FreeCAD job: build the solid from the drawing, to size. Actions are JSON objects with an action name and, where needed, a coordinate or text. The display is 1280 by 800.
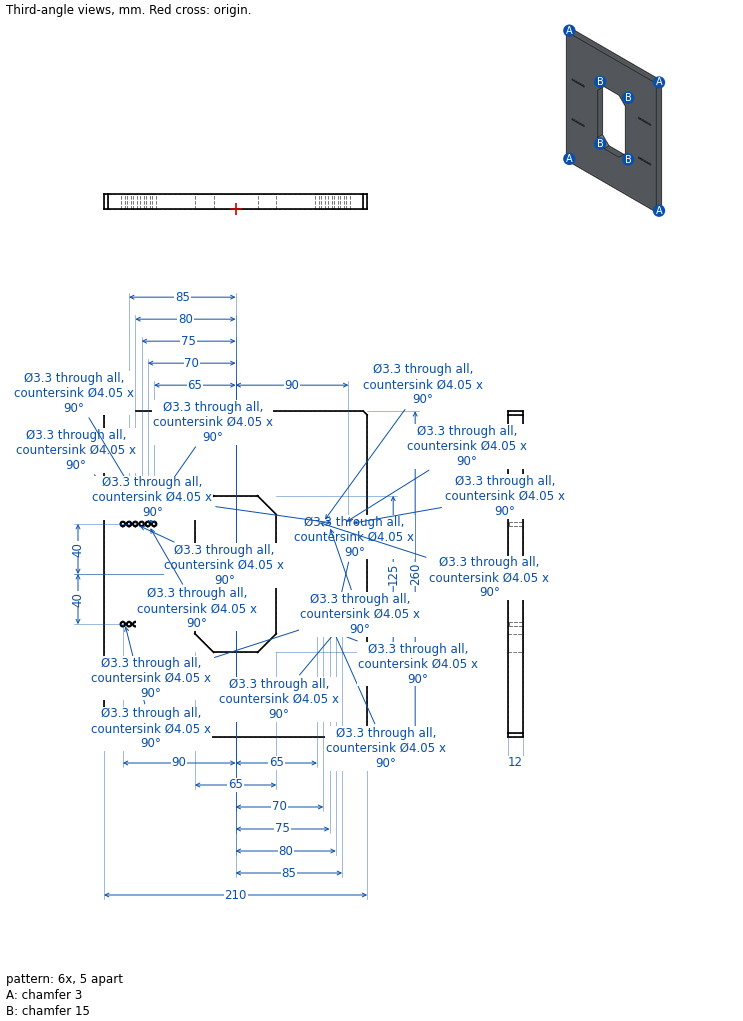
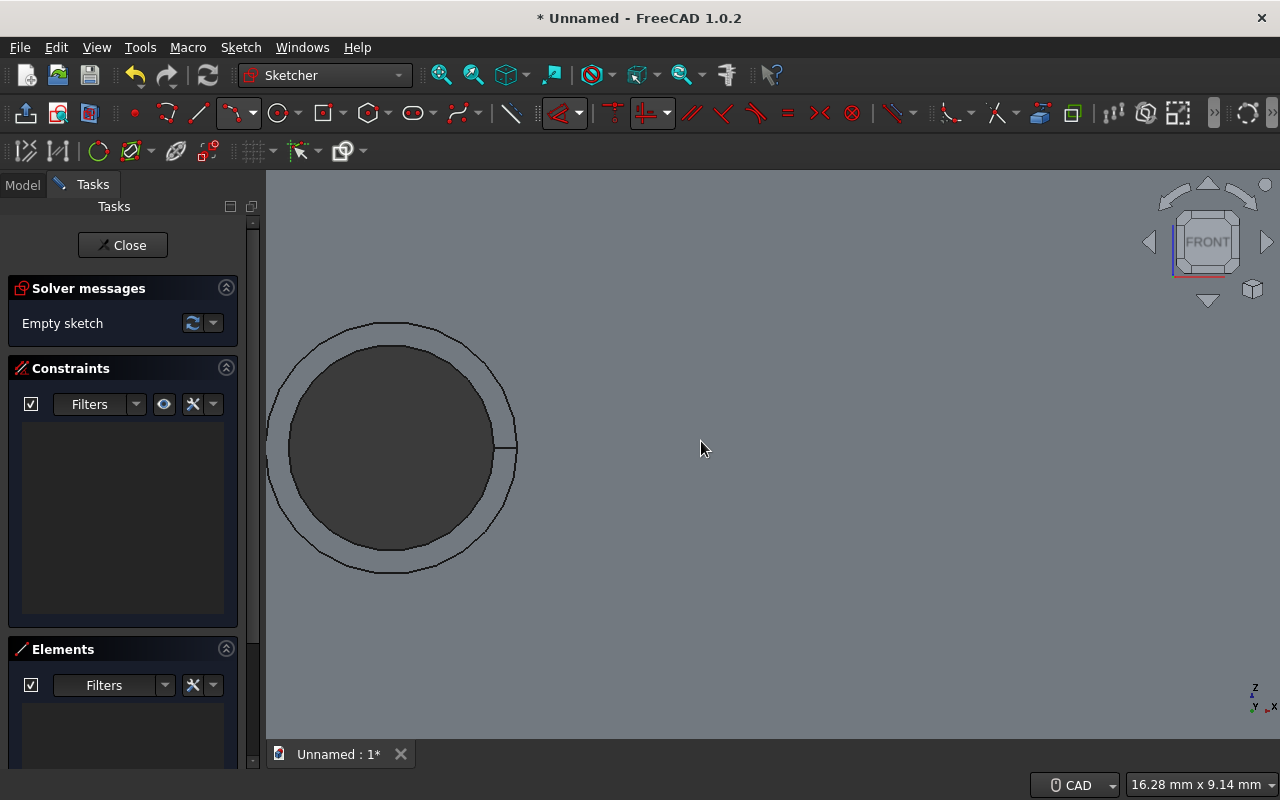
{"action": "left_click", "coordinate": [278, 114]}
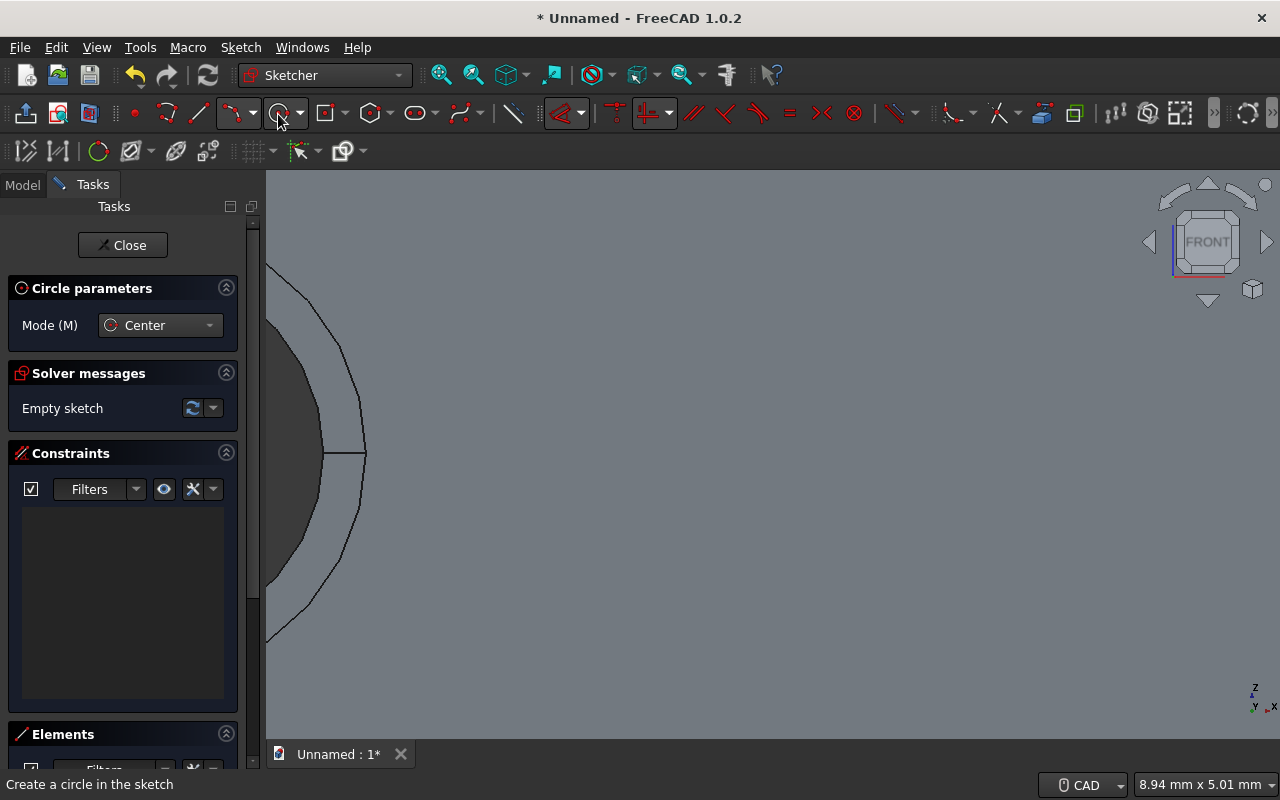
{"action": "left_click", "coordinate": [703, 453]}
{"action": "mouse_move", "coordinate": [836, 321]}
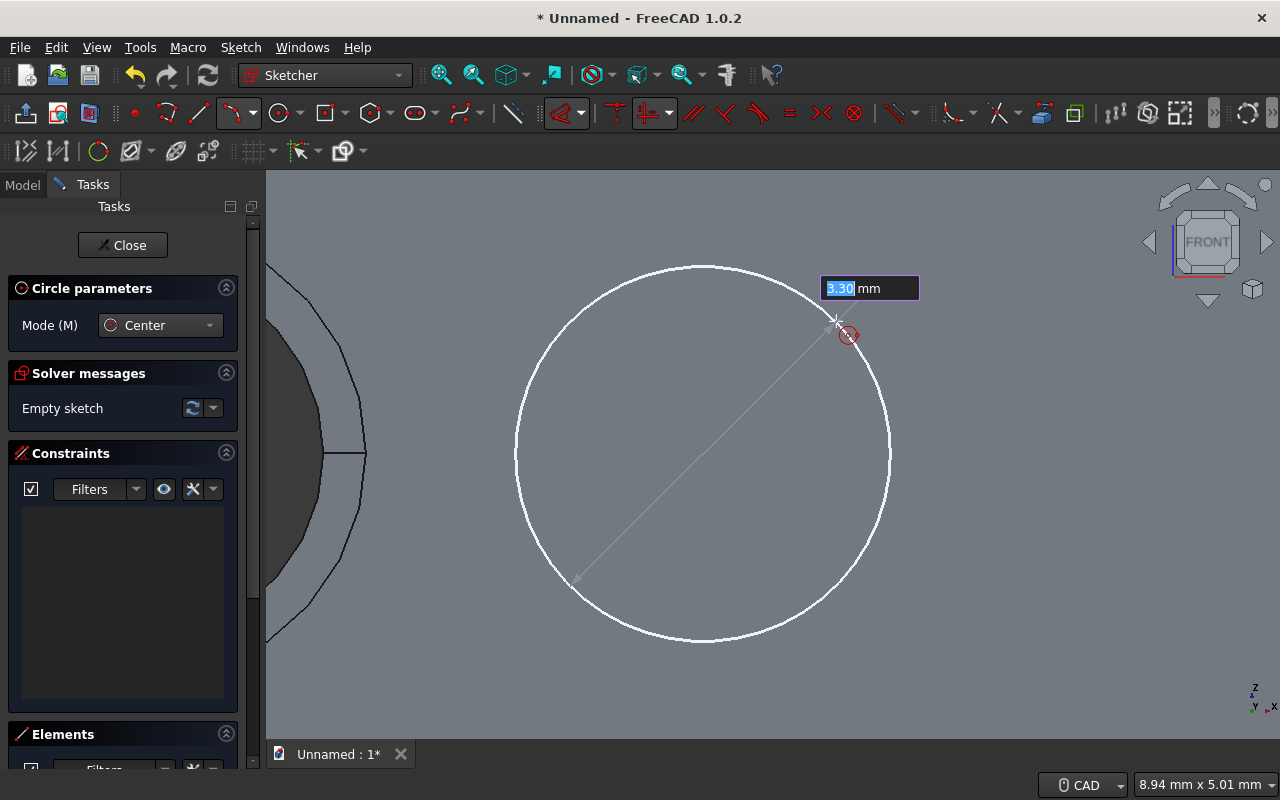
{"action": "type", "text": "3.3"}
{"action": "key", "text": "Return"}
{"action": "key", "text": "Escape"}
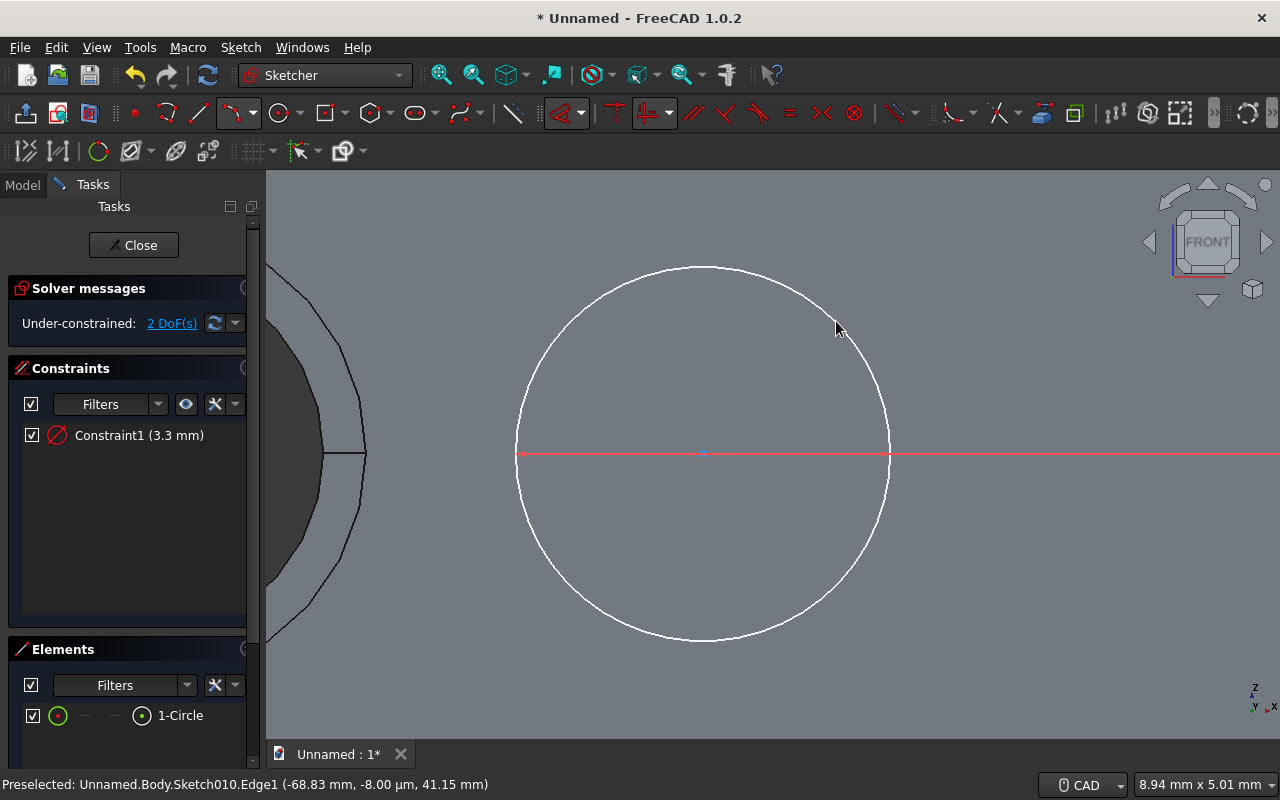
{"action": "left_click", "coordinate": [703, 454]}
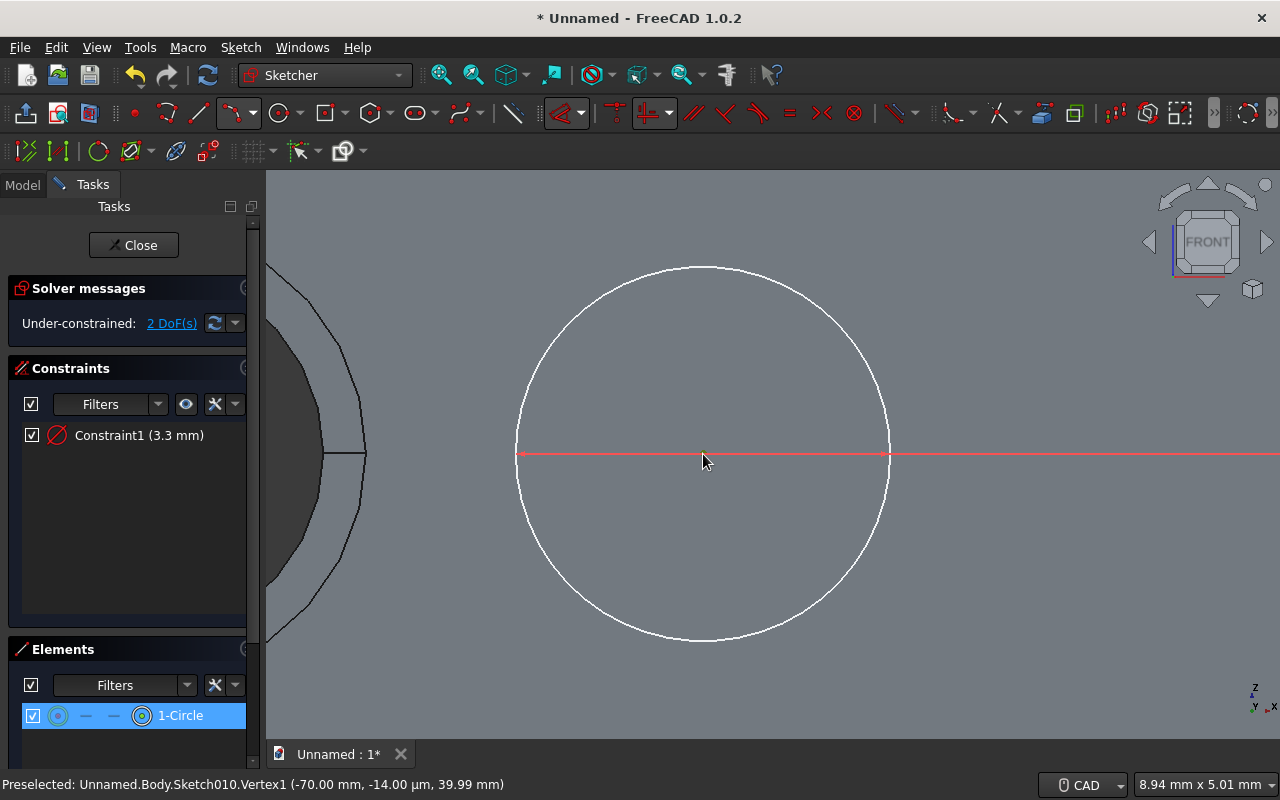
{"action": "left_click", "coordinate": [584, 114]}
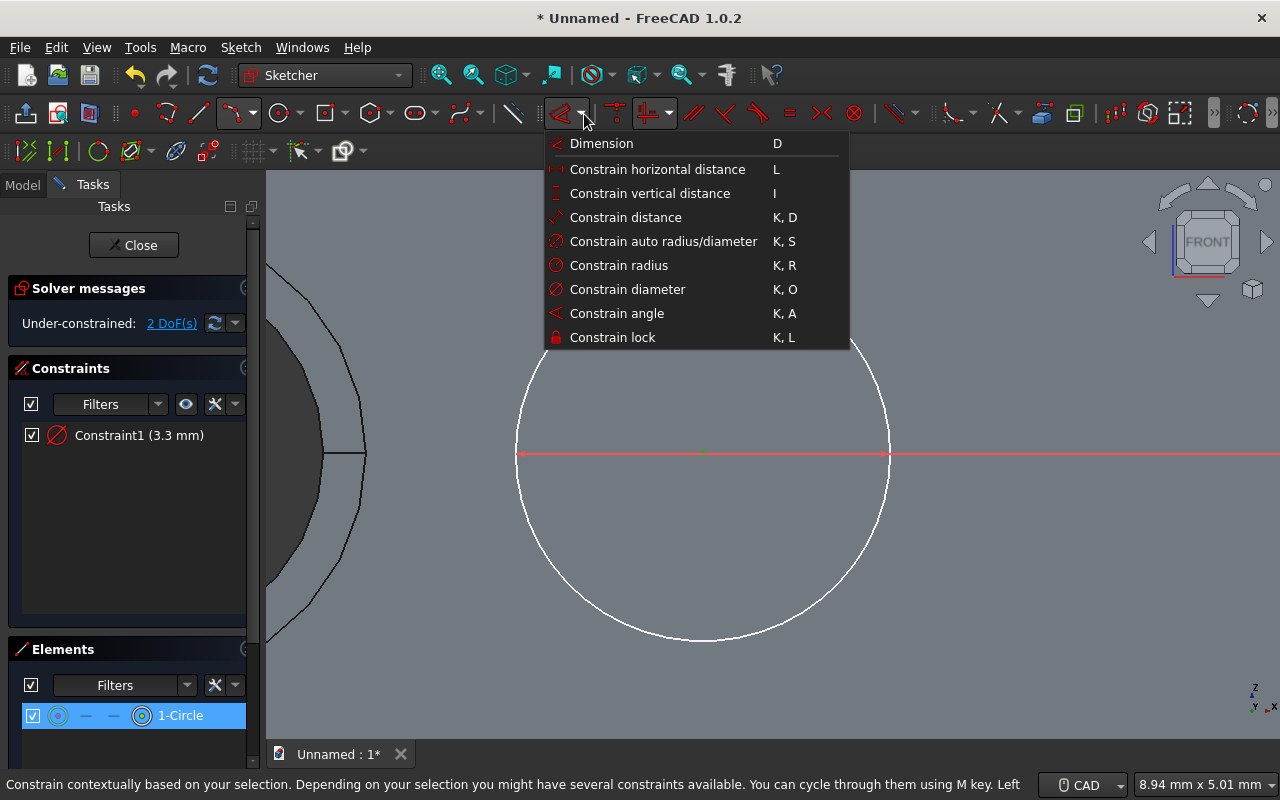
{"action": "left_click", "coordinate": [697, 169]}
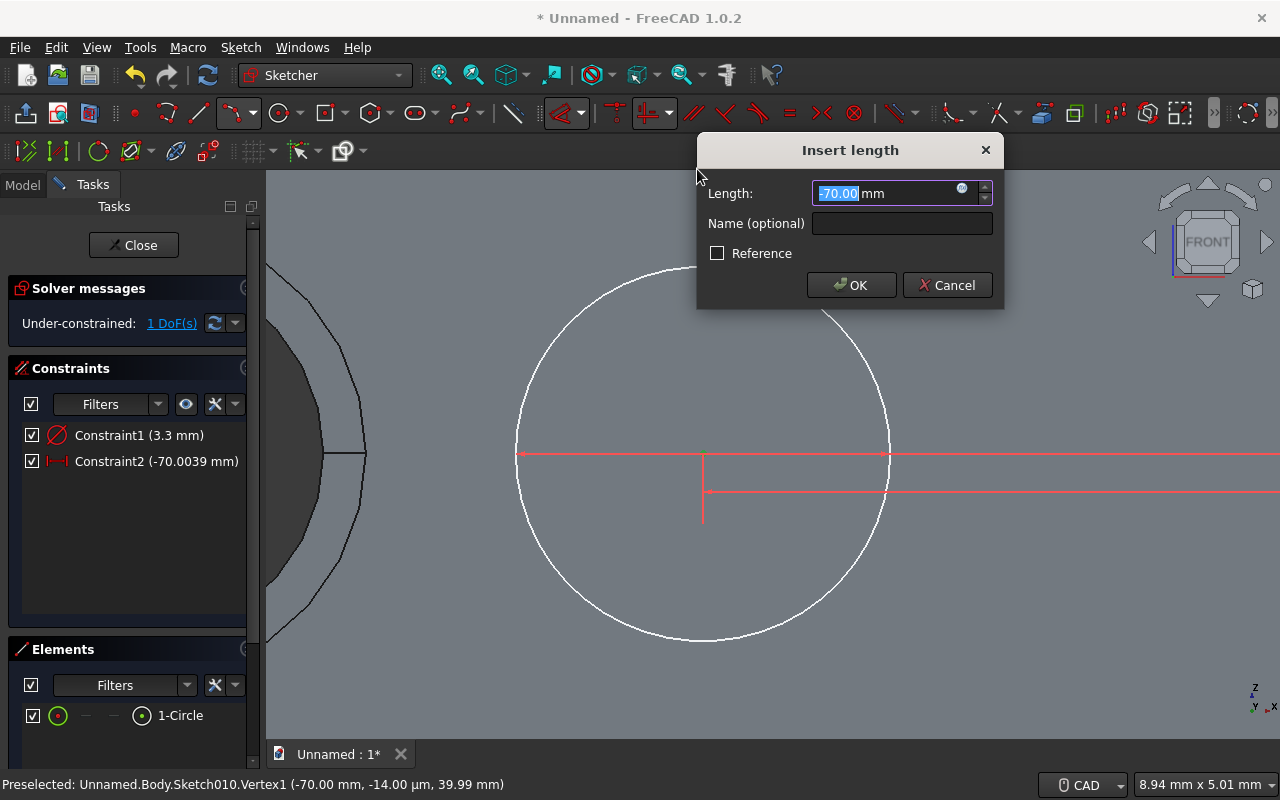
{"action": "type", "text": "-70"}
{"action": "key", "text": "Return"}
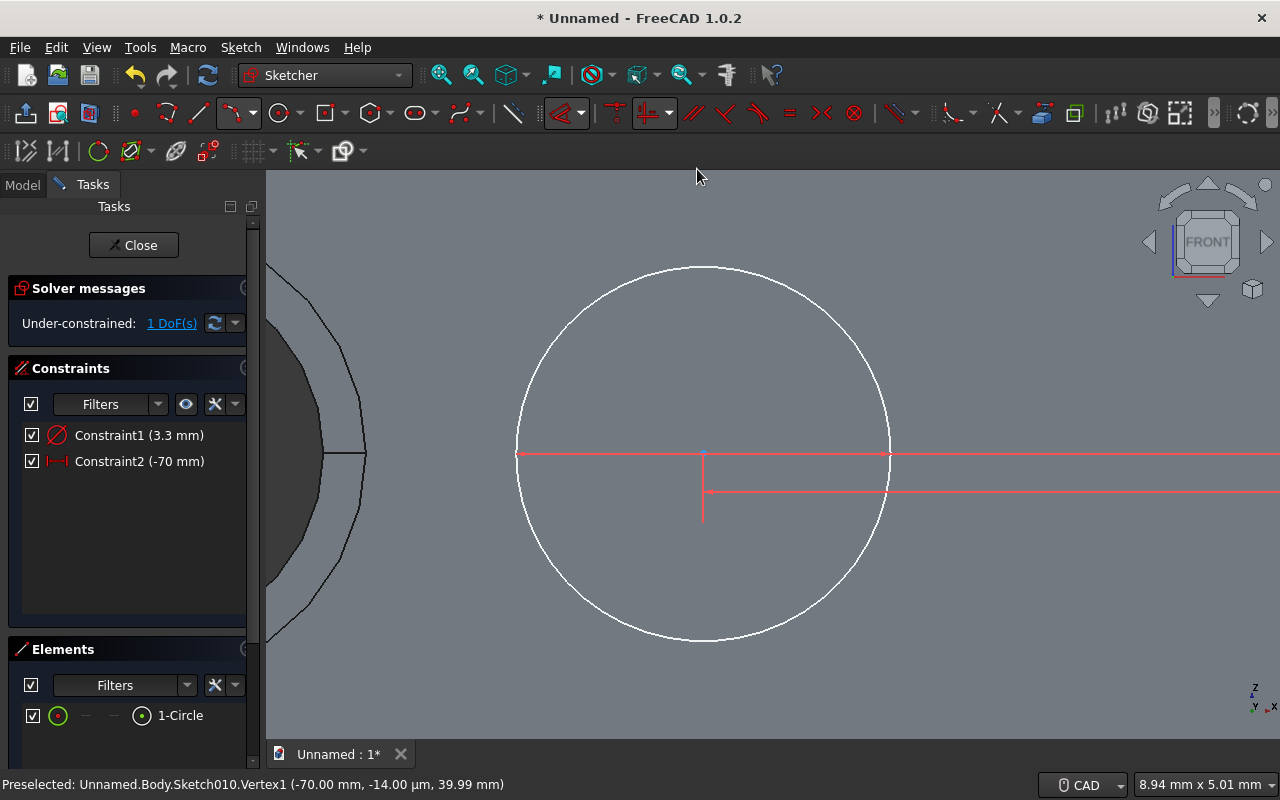
{"action": "left_click", "coordinate": [703, 454]}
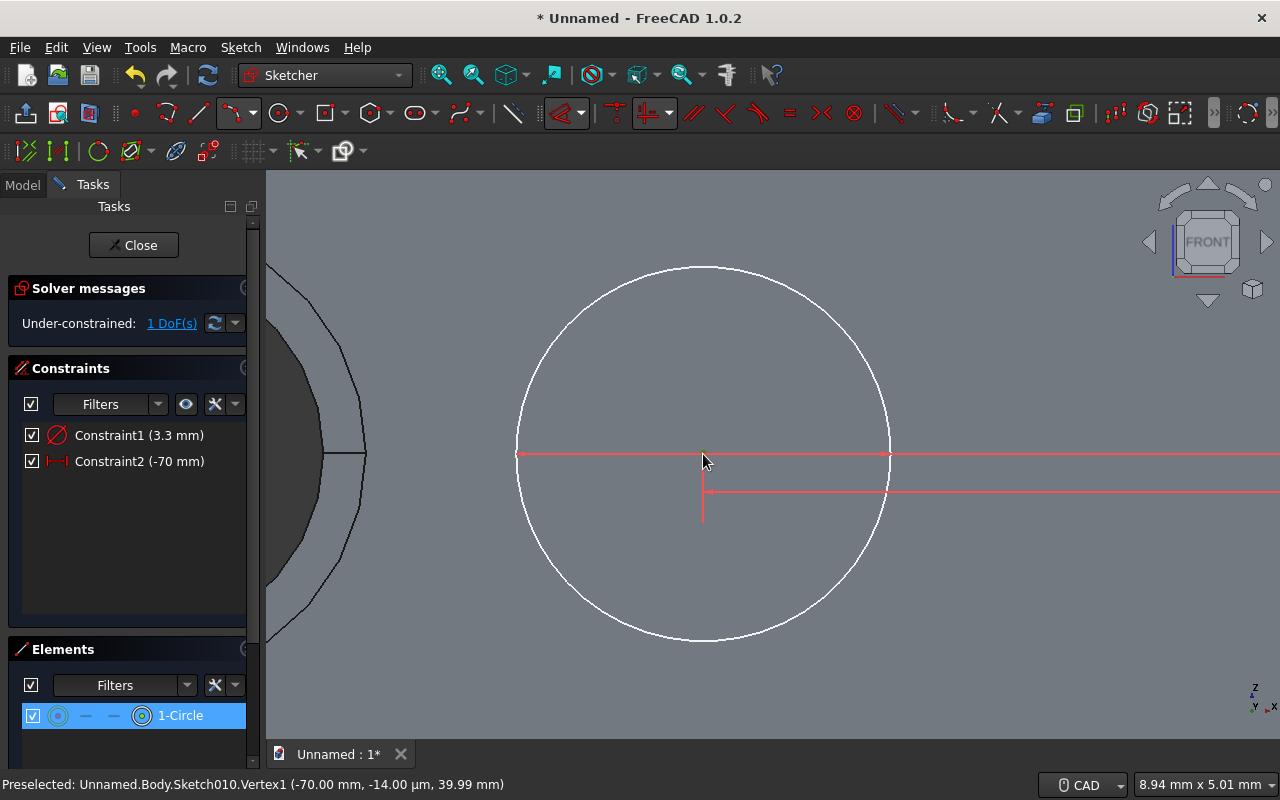
{"action": "key", "text": "i"}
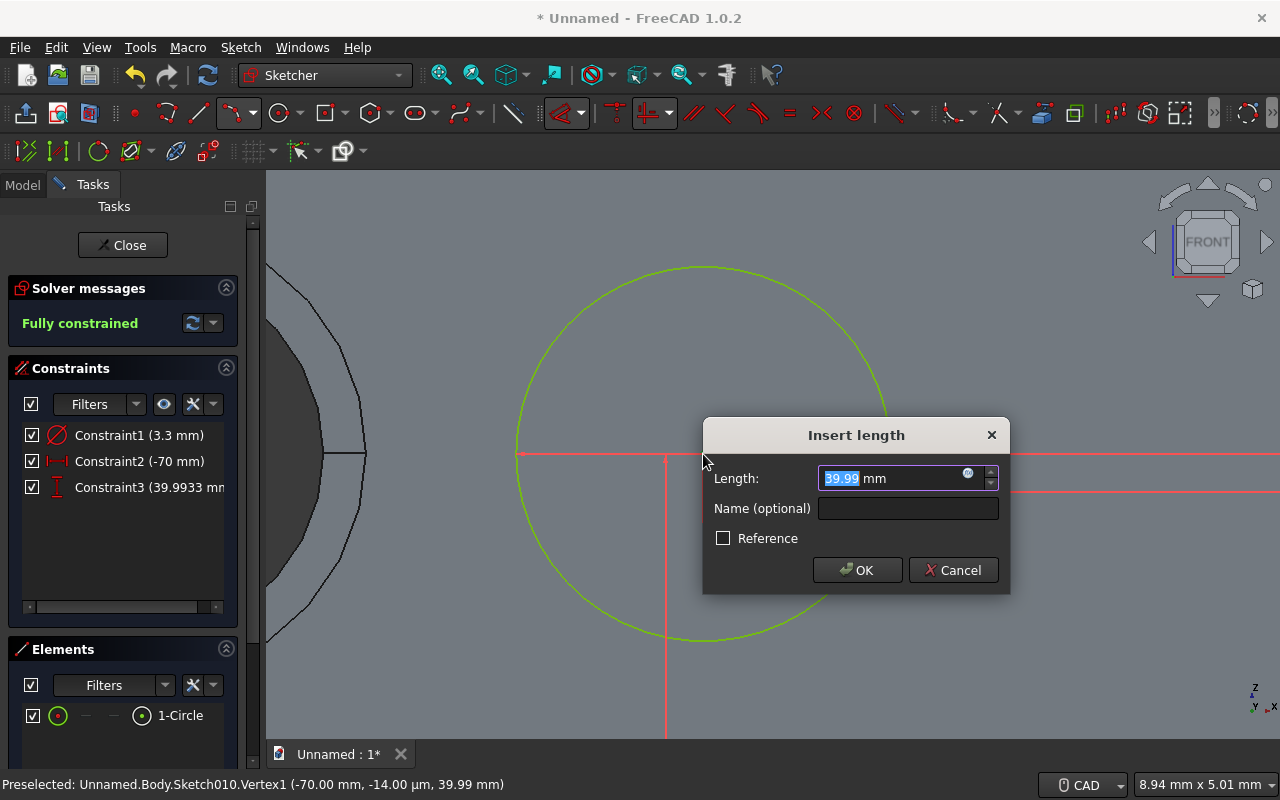
{"action": "type", "text": "40"}
{"action": "key", "text": "Return"}